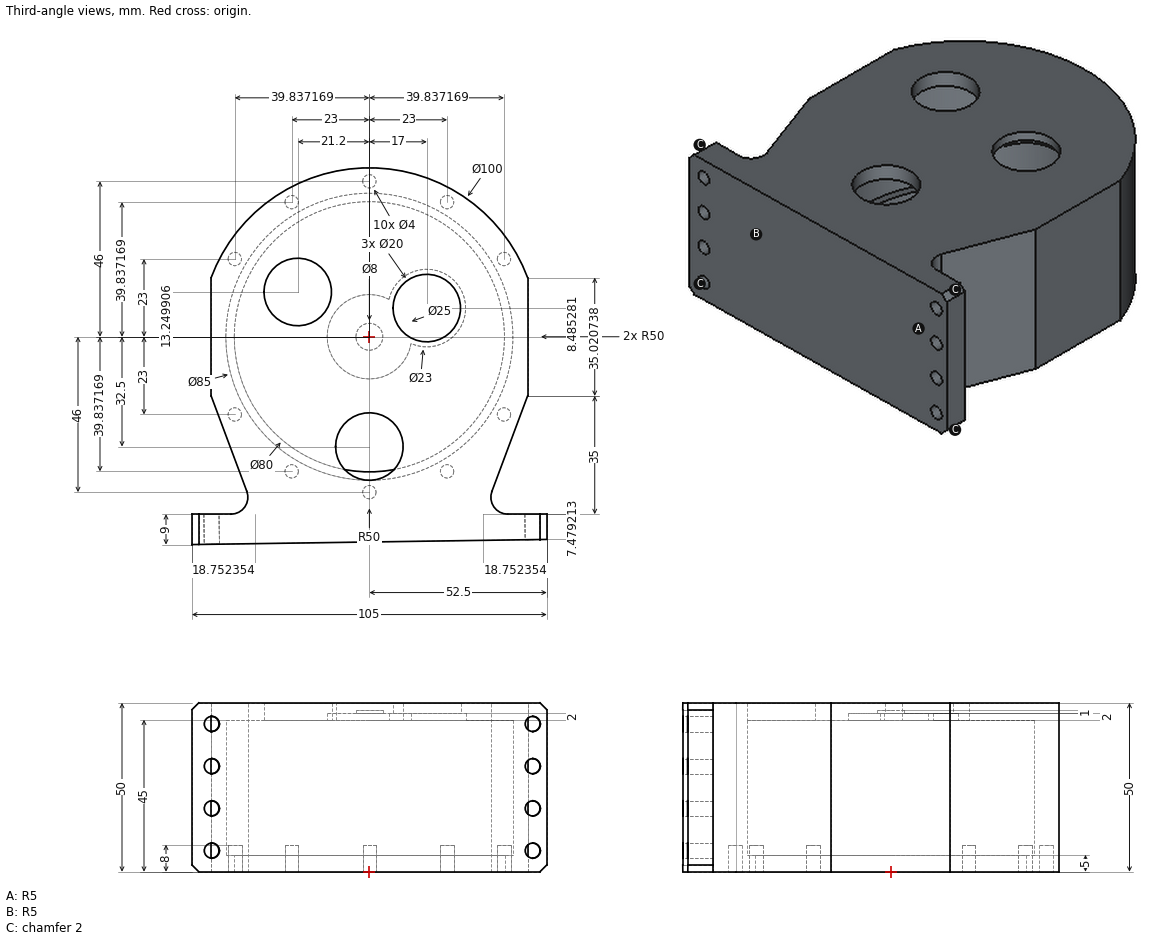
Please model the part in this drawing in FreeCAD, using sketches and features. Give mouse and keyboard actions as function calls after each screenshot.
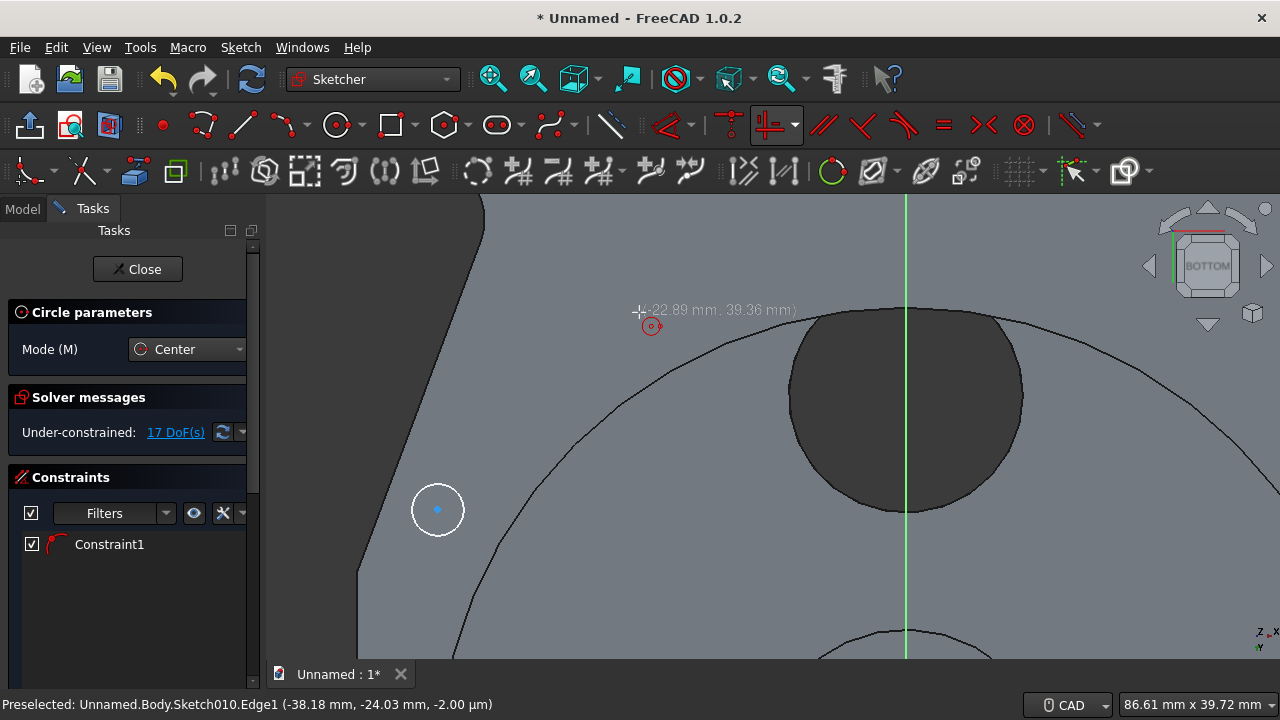
scroll(639, 312, down, 7)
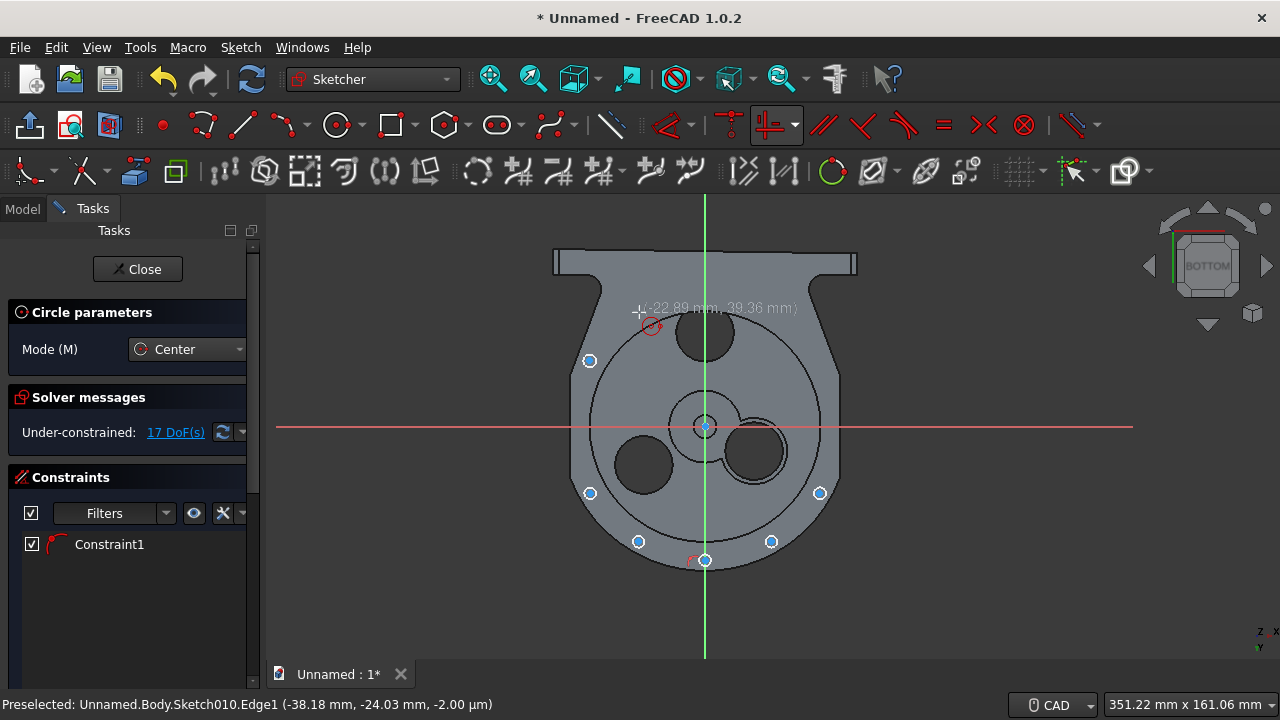
click(639, 312)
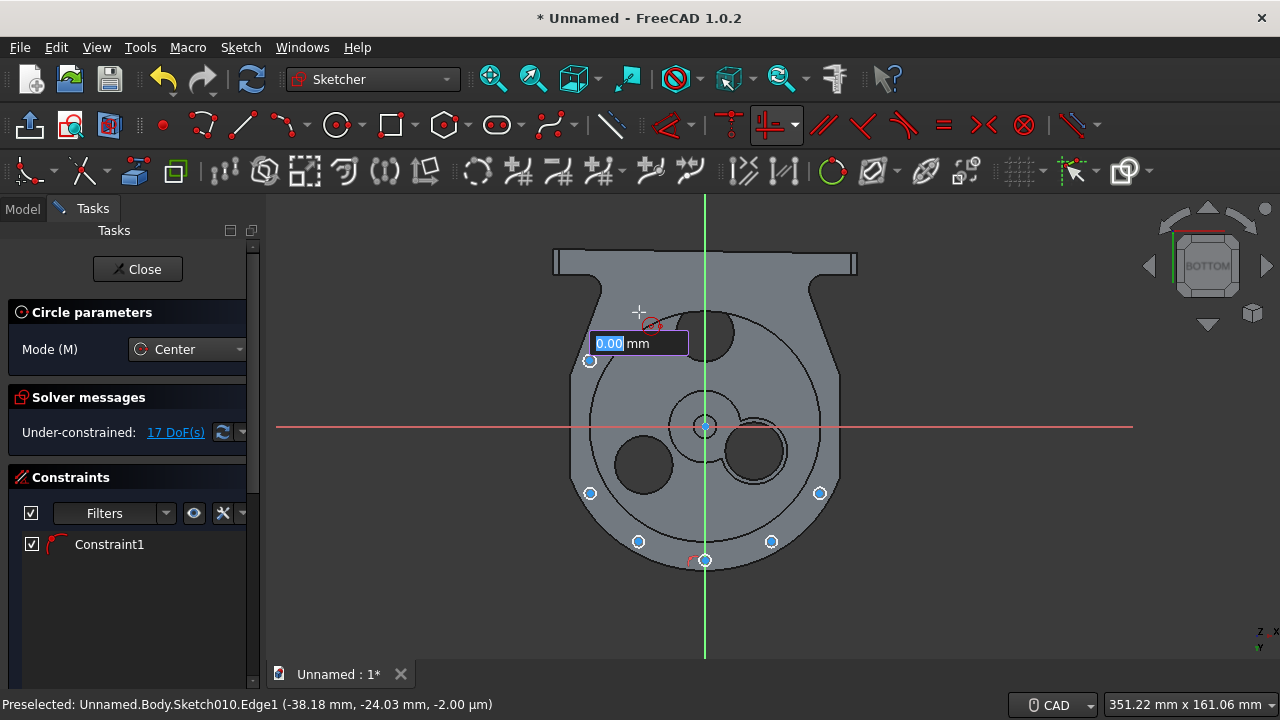
scroll(643, 308, up, 6)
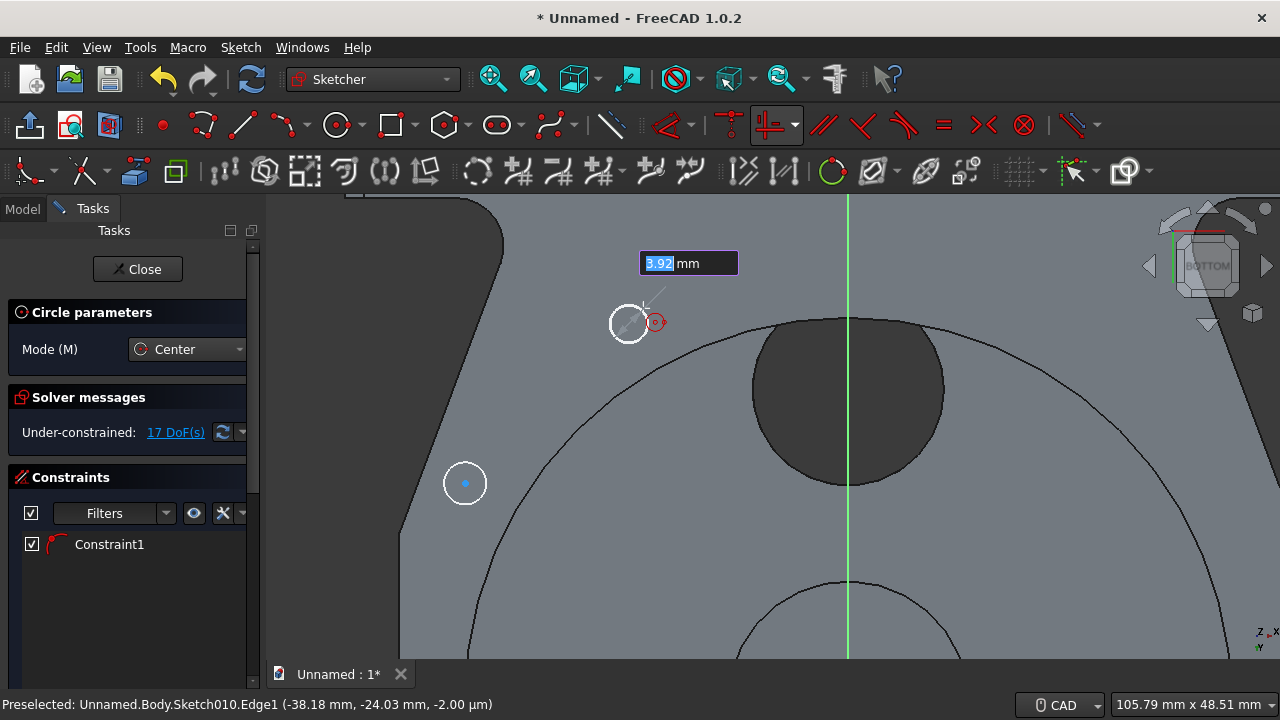
click(641, 306)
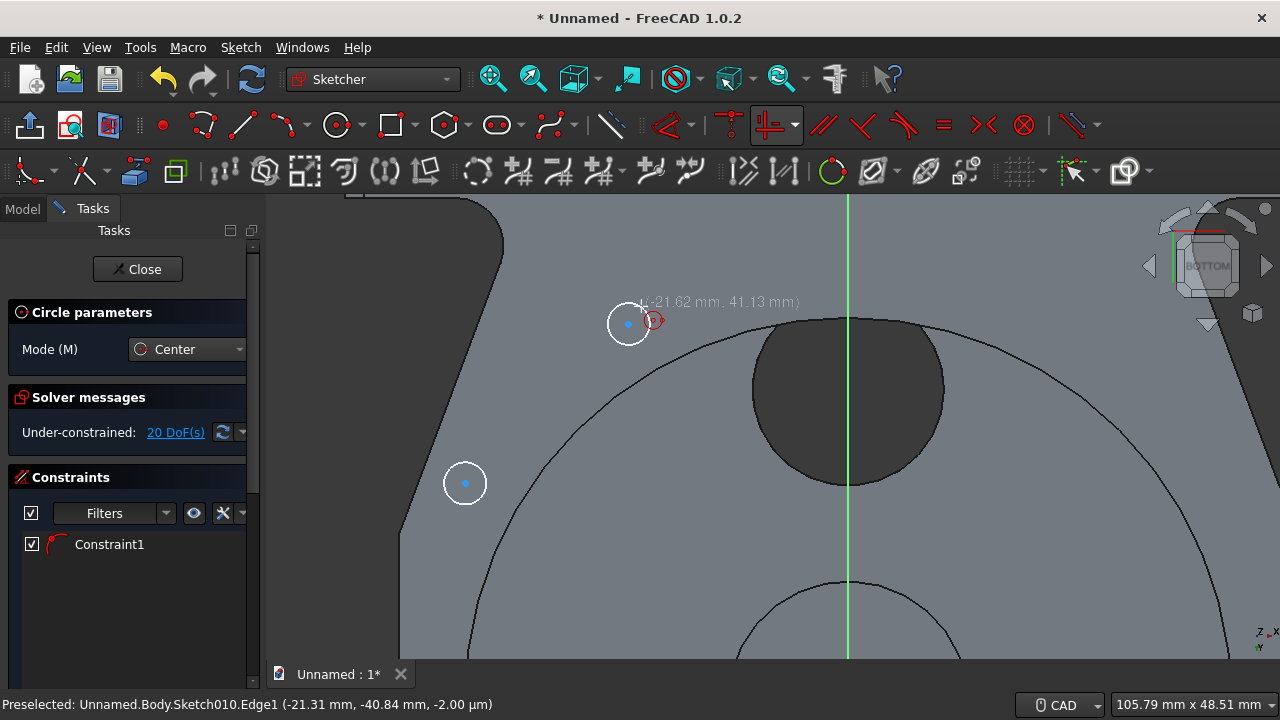
click(848, 260)
click(866, 254)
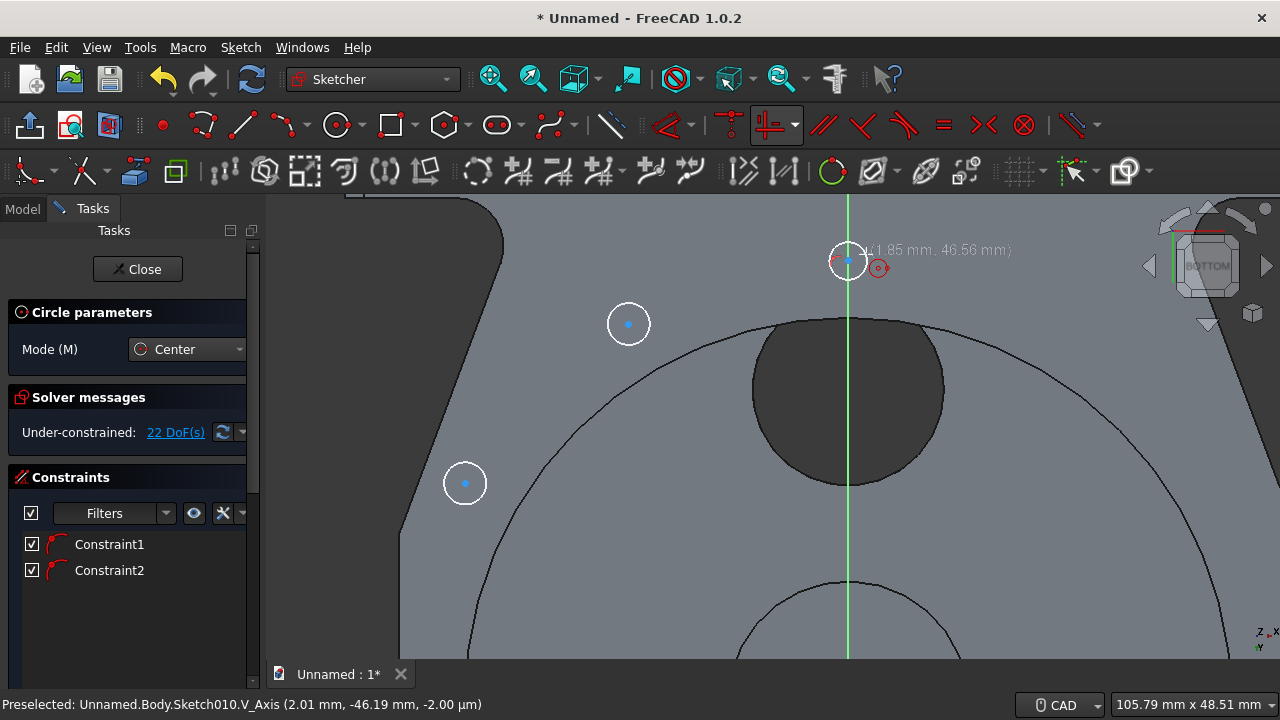
click(1069, 319)
click(1082, 306)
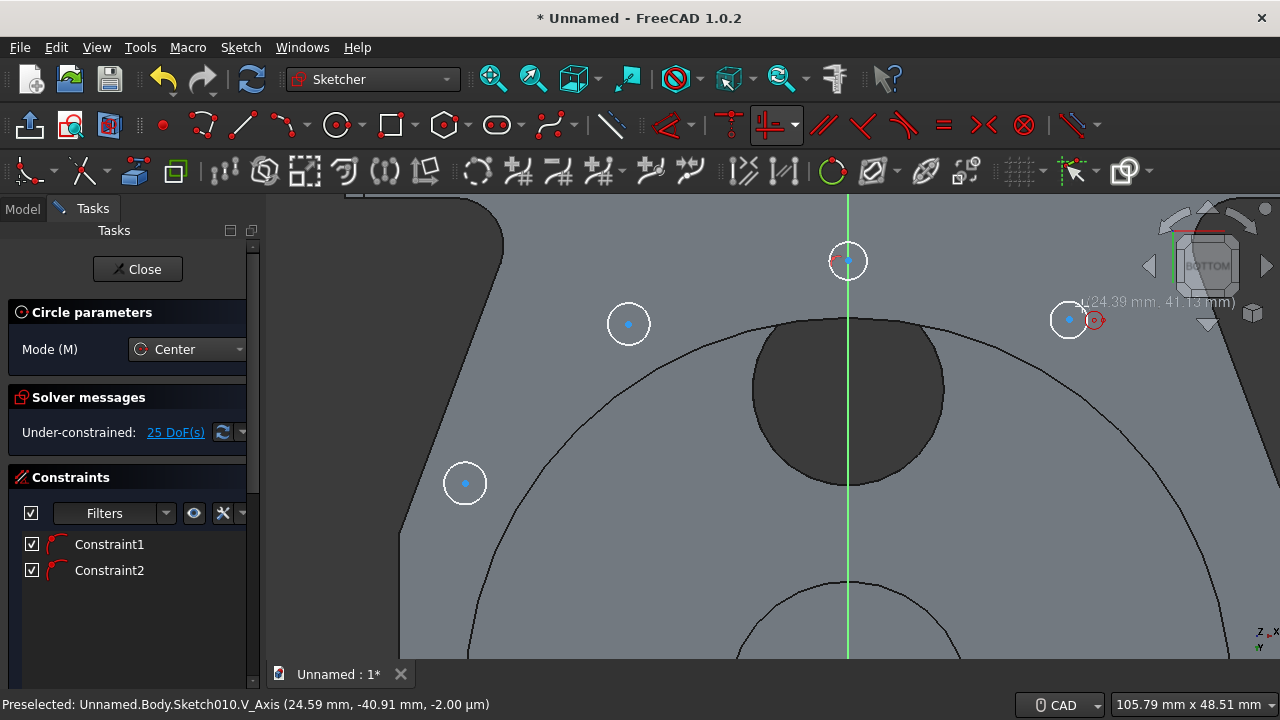
scroll(643, 308, down, 6)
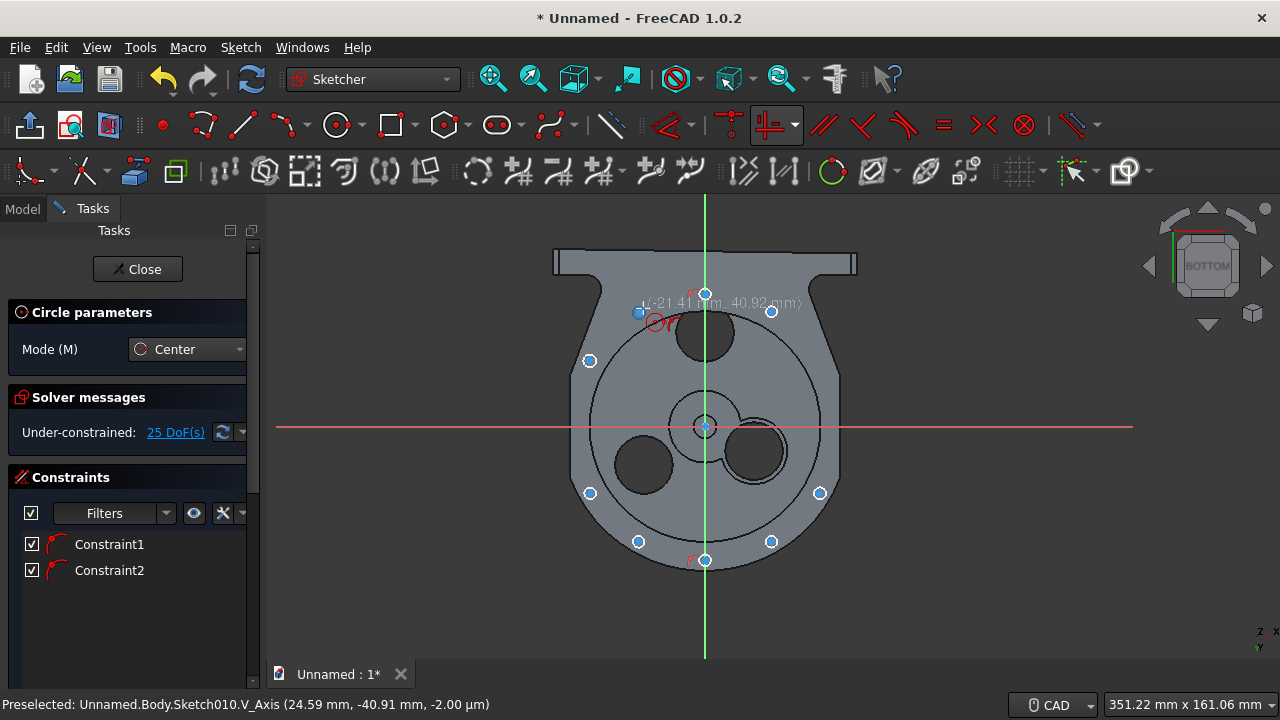
scroll(820, 360, up, 7)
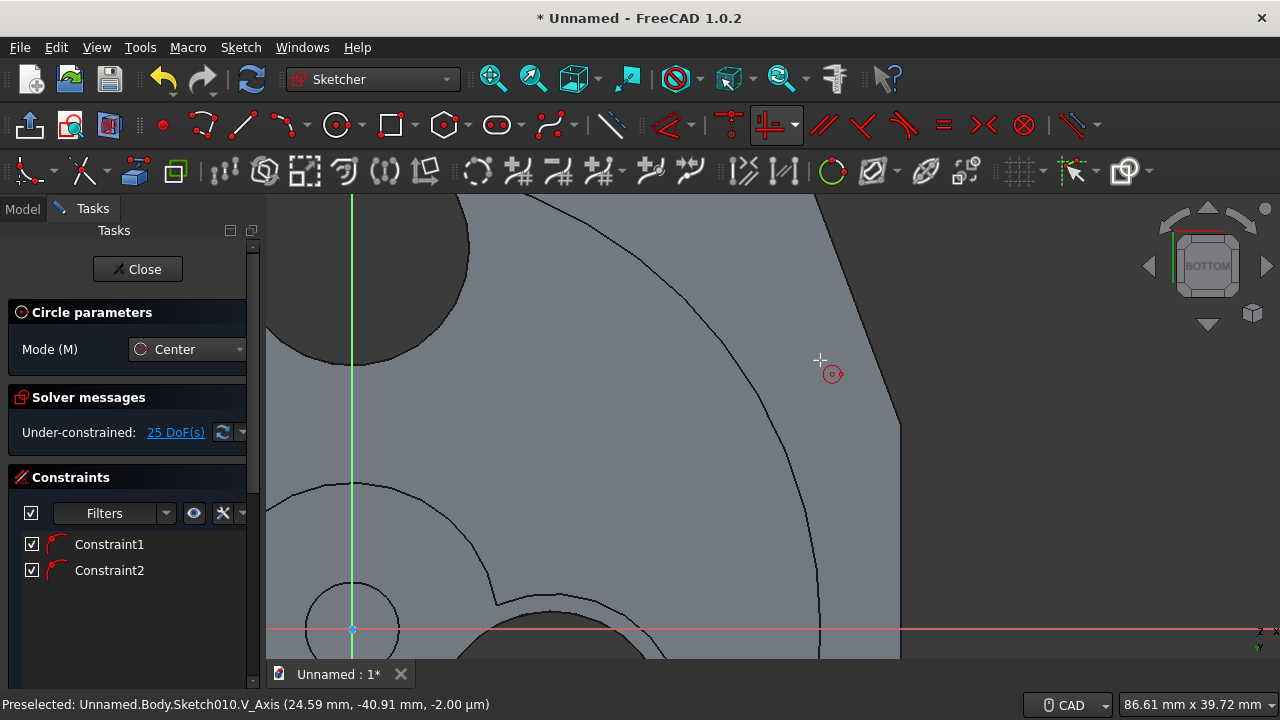
scroll(820, 360, down, 7)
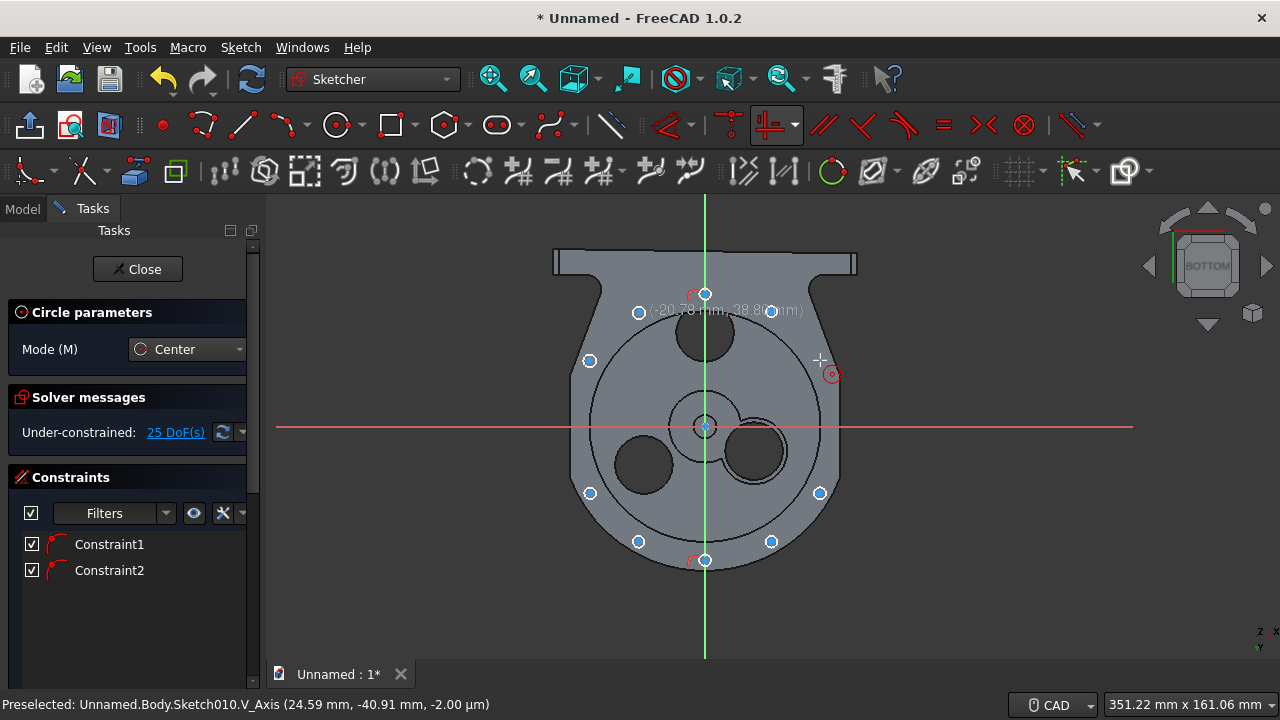
click(820, 360)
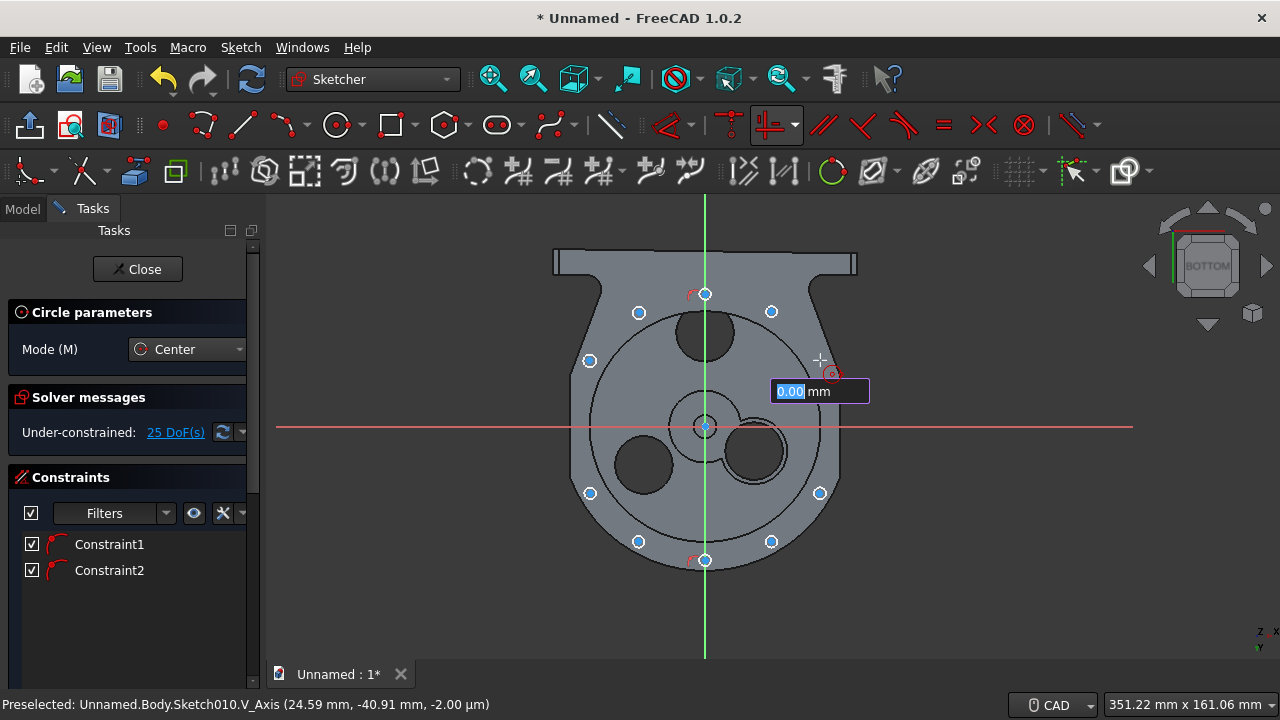
scroll(824, 356, up, 6)